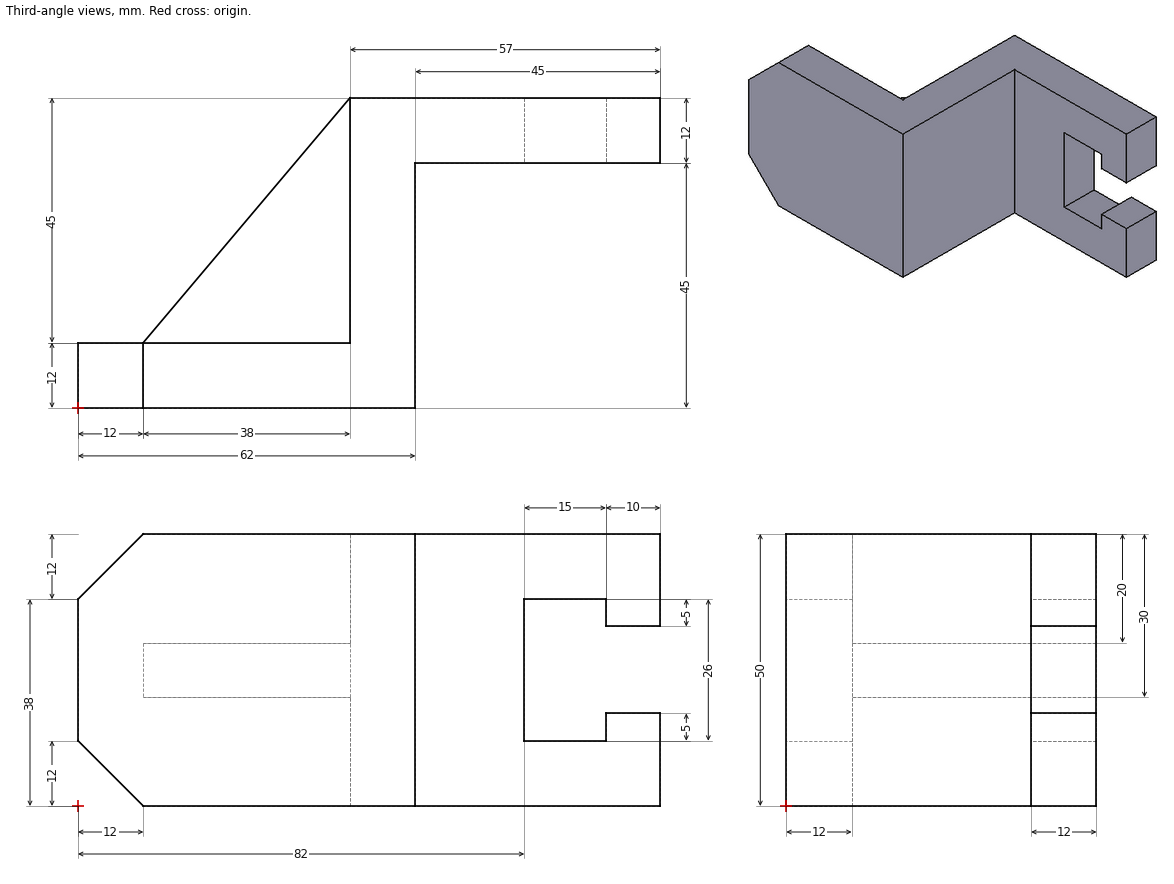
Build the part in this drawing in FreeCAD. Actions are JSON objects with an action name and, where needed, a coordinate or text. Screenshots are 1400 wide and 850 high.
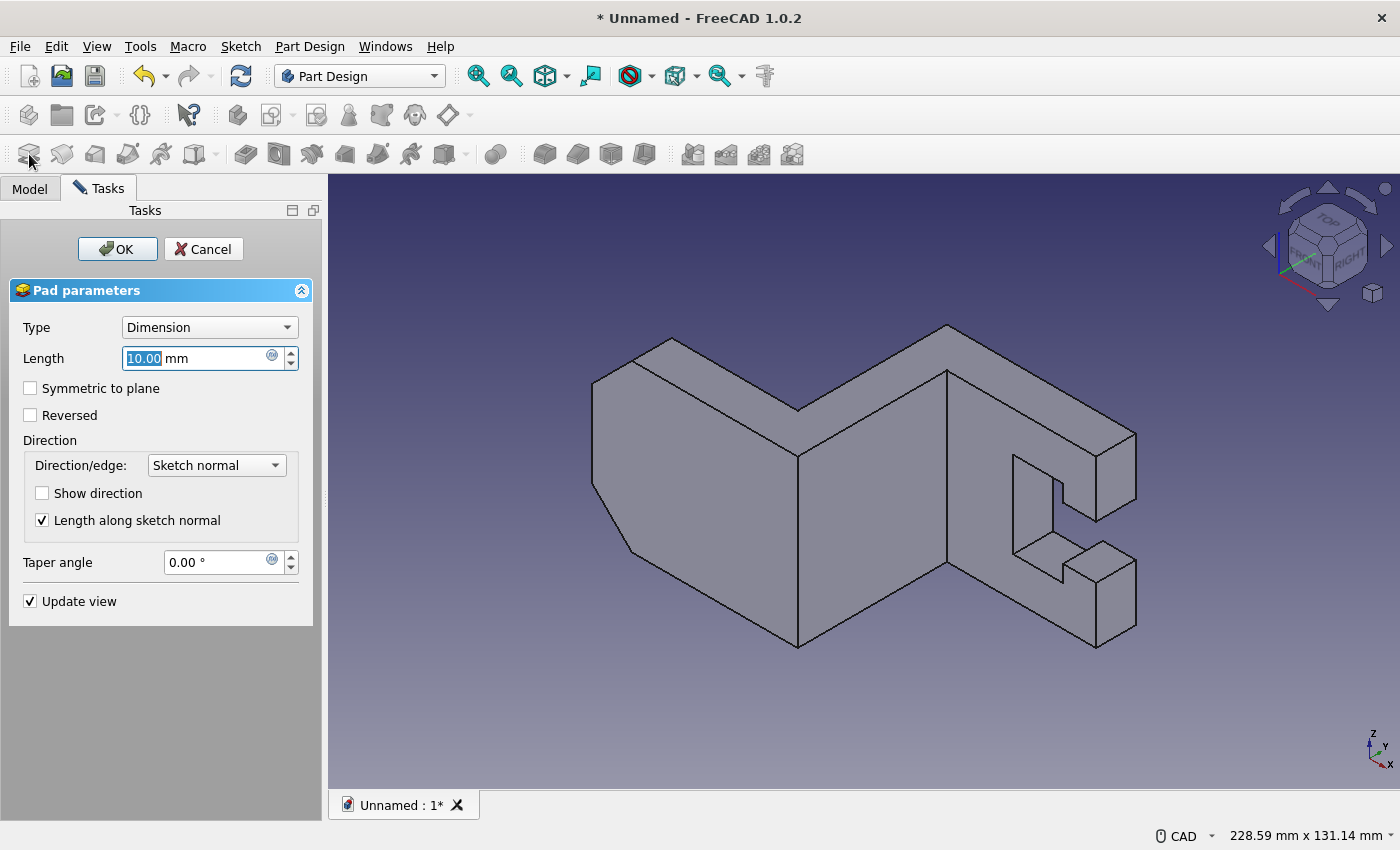
{"action": "type", "text": "30"}
{"action": "key", "text": "Tab"}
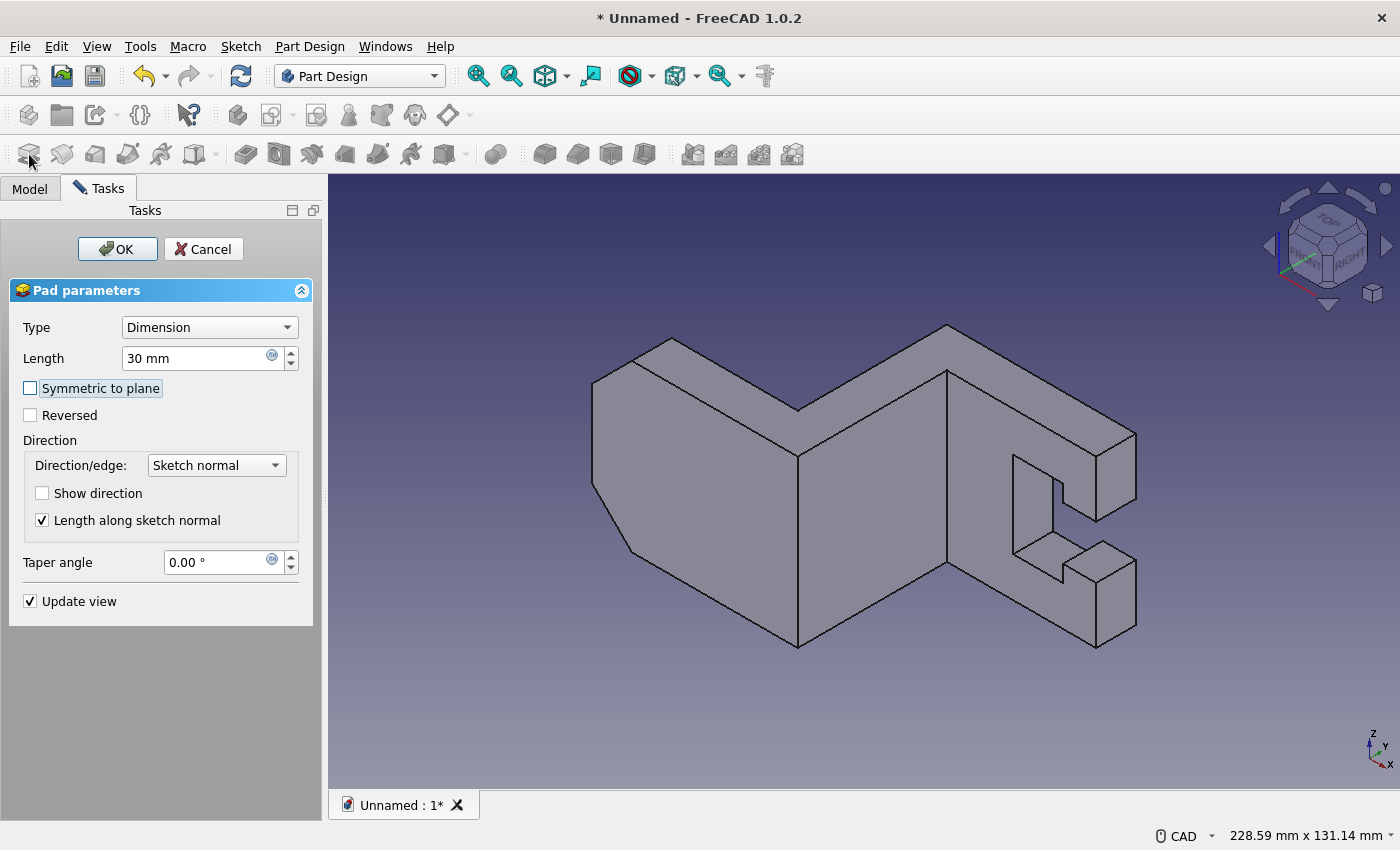
{"action": "left_click", "coordinate": [31, 415]}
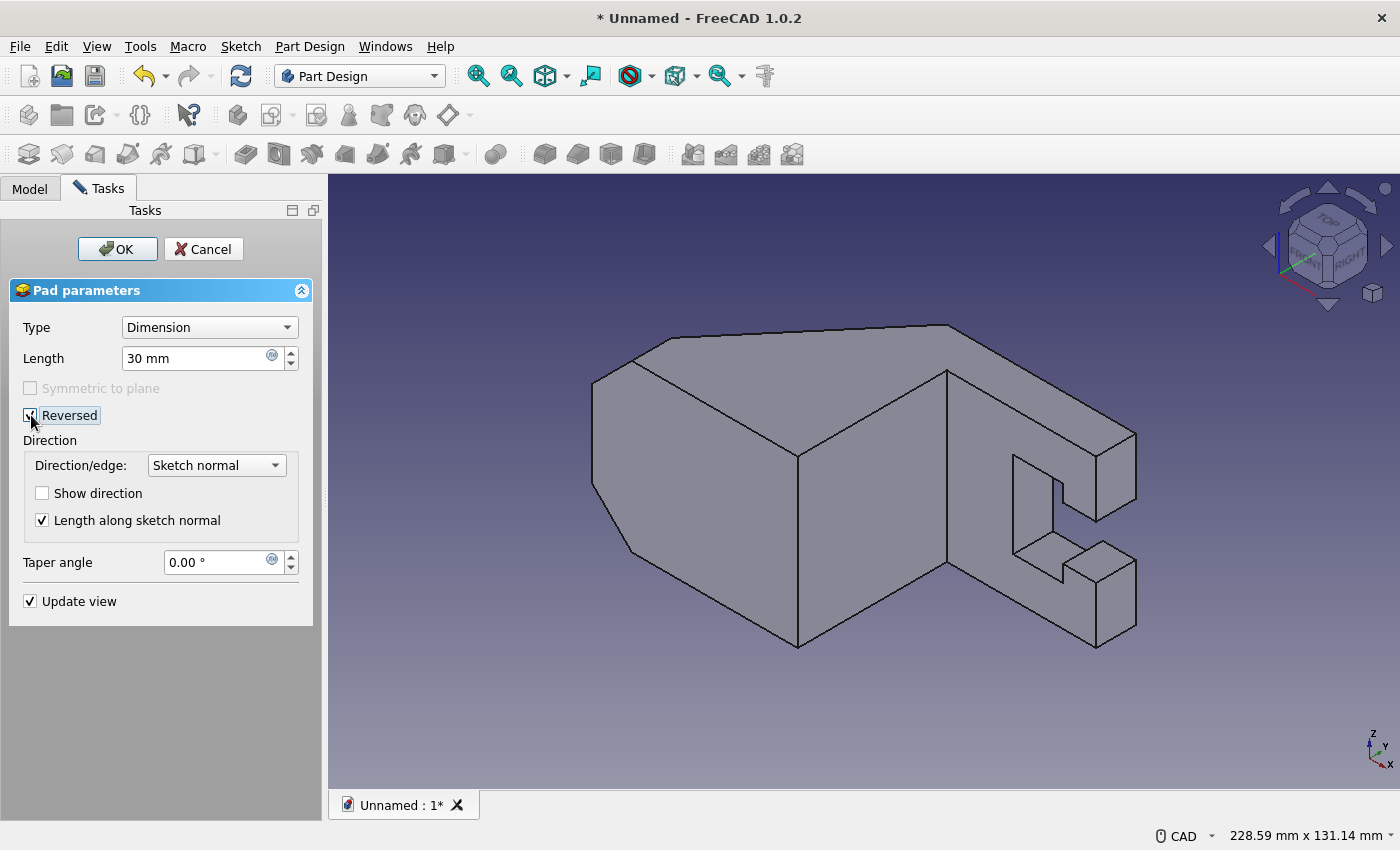
{"action": "left_click", "coordinate": [118, 249]}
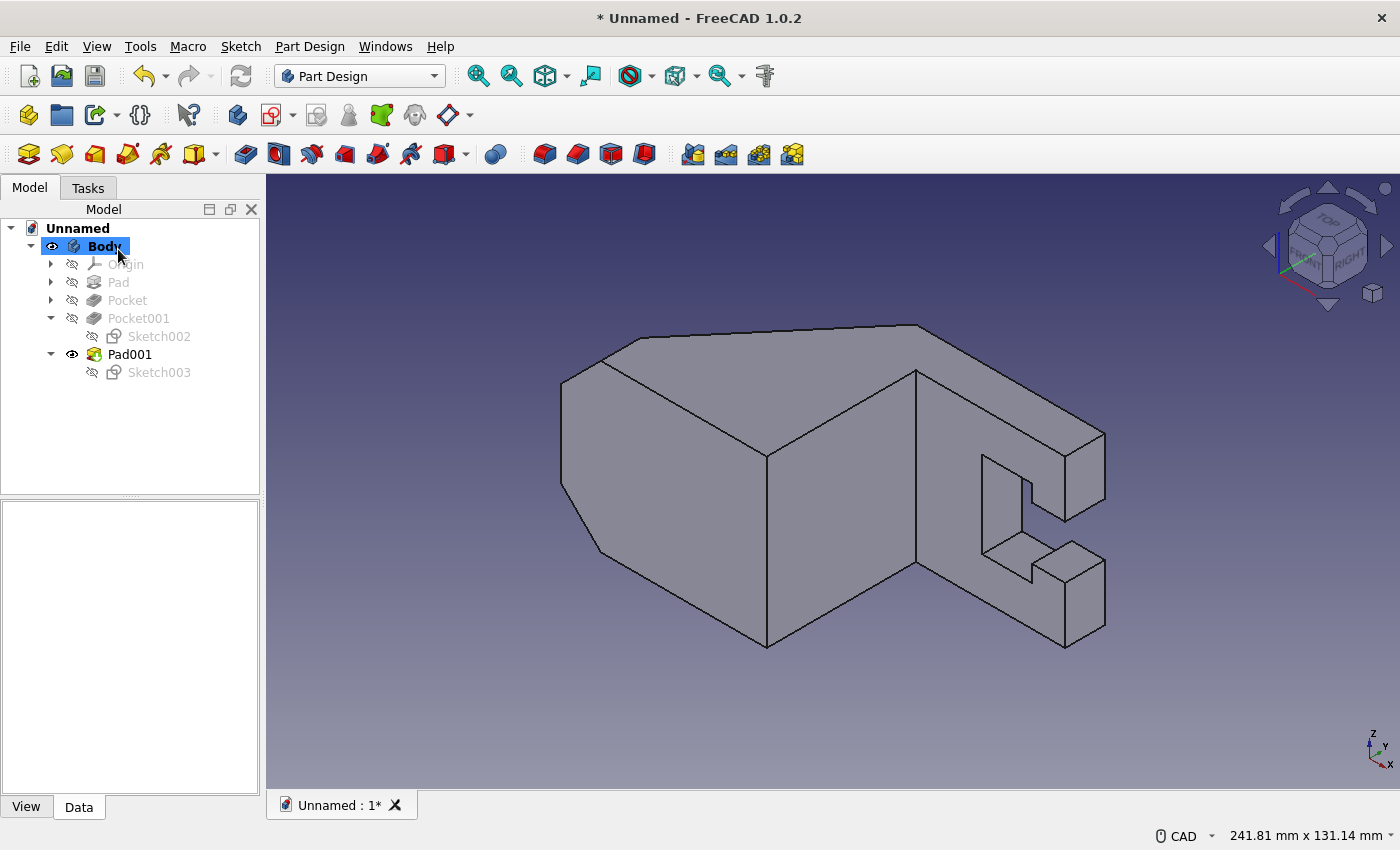
{"action": "left_click", "coordinate": [781, 386]}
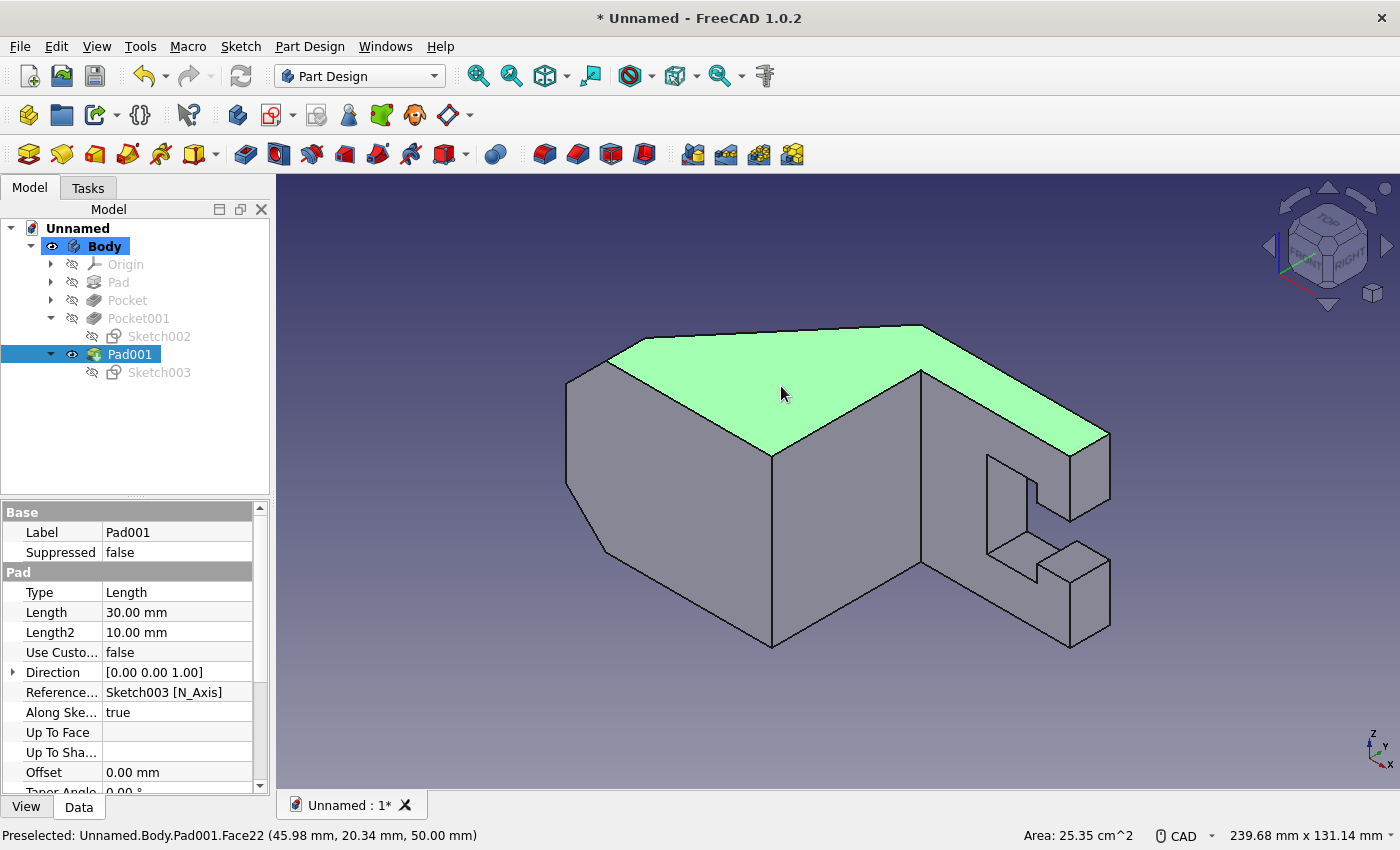
{"action": "left_click", "coordinate": [270, 116]}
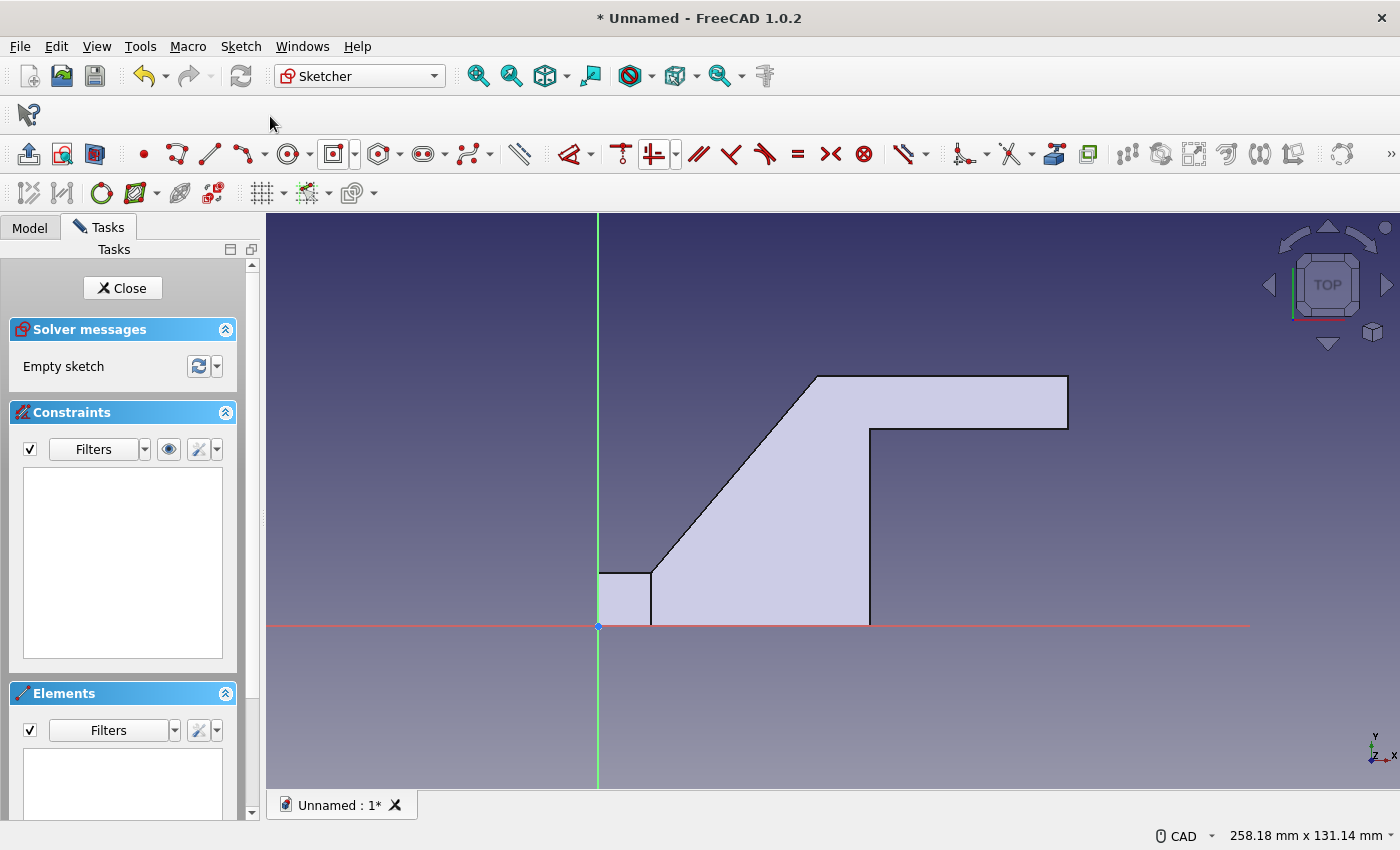
{"action": "scroll", "coordinate": [593, 501], "scroll_direction": "up", "scroll_amount": 2}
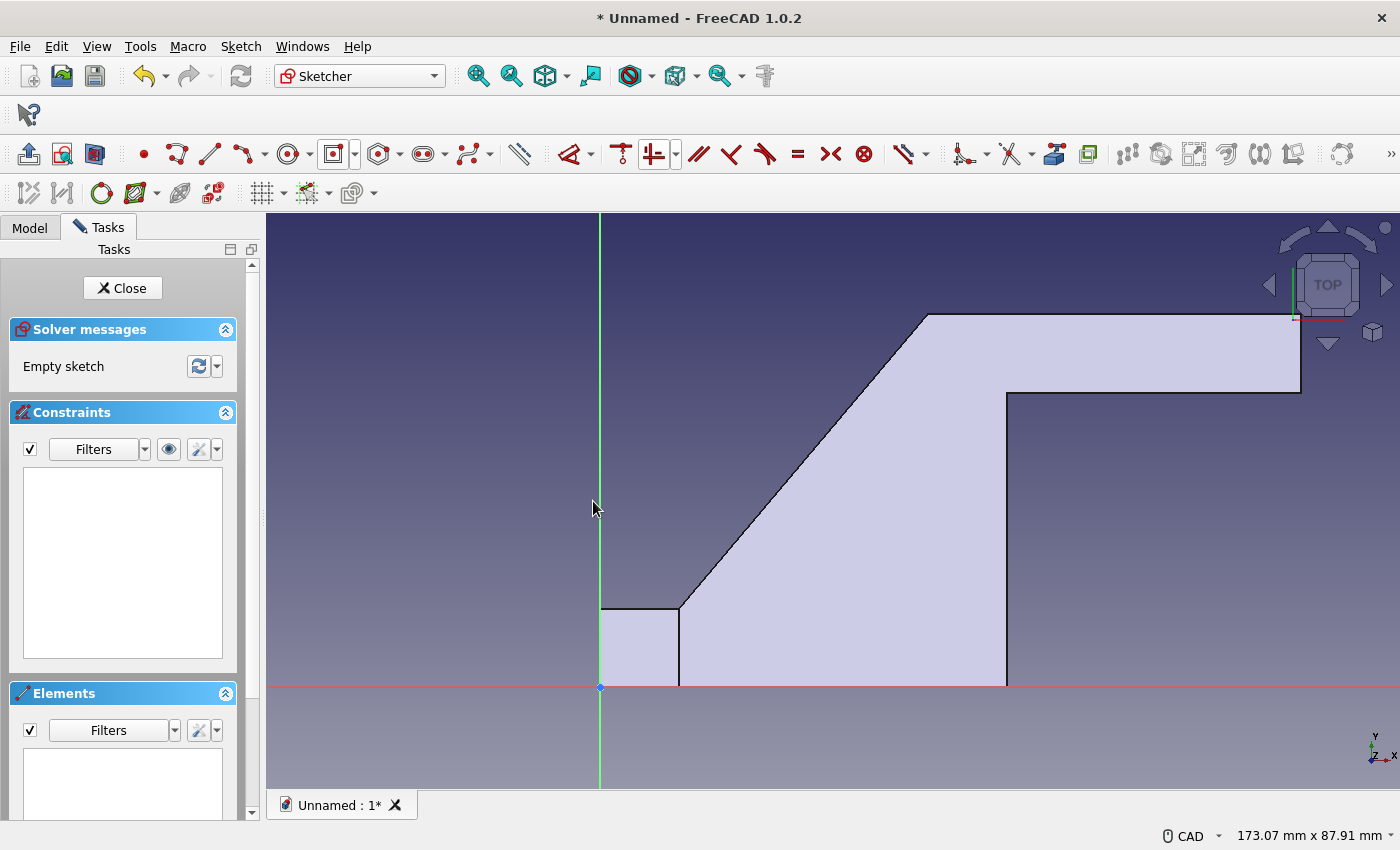
{"action": "left_click", "coordinate": [177, 154]}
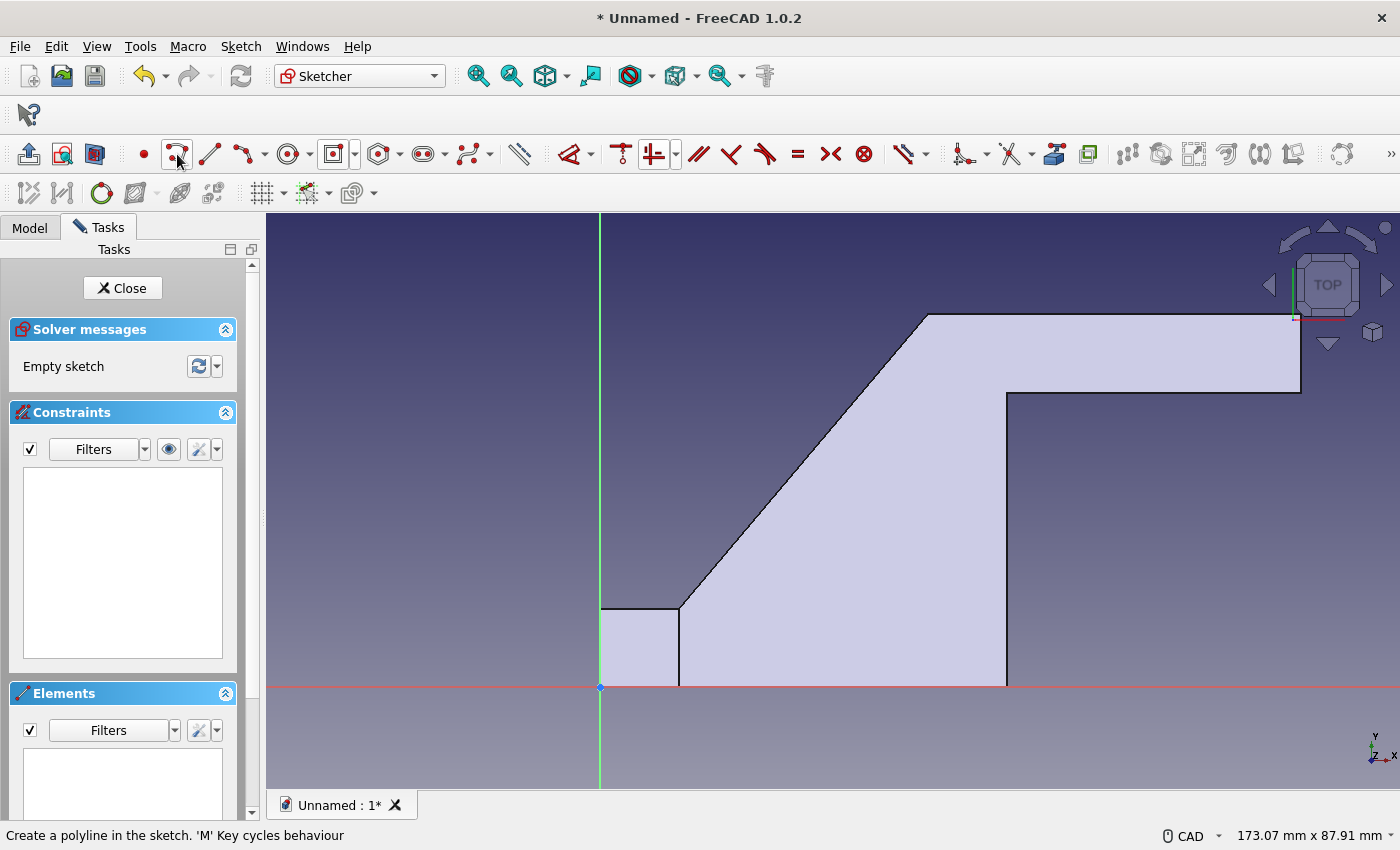
{"action": "left_click", "coordinate": [679, 609]}
{"action": "left_click", "coordinate": [928, 609]}
{"action": "left_click", "coordinate": [928, 314]}
{"action": "left_click", "coordinate": [679, 610]}
{"action": "key", "text": "Escape"}
{"action": "key", "text": "Escape"}